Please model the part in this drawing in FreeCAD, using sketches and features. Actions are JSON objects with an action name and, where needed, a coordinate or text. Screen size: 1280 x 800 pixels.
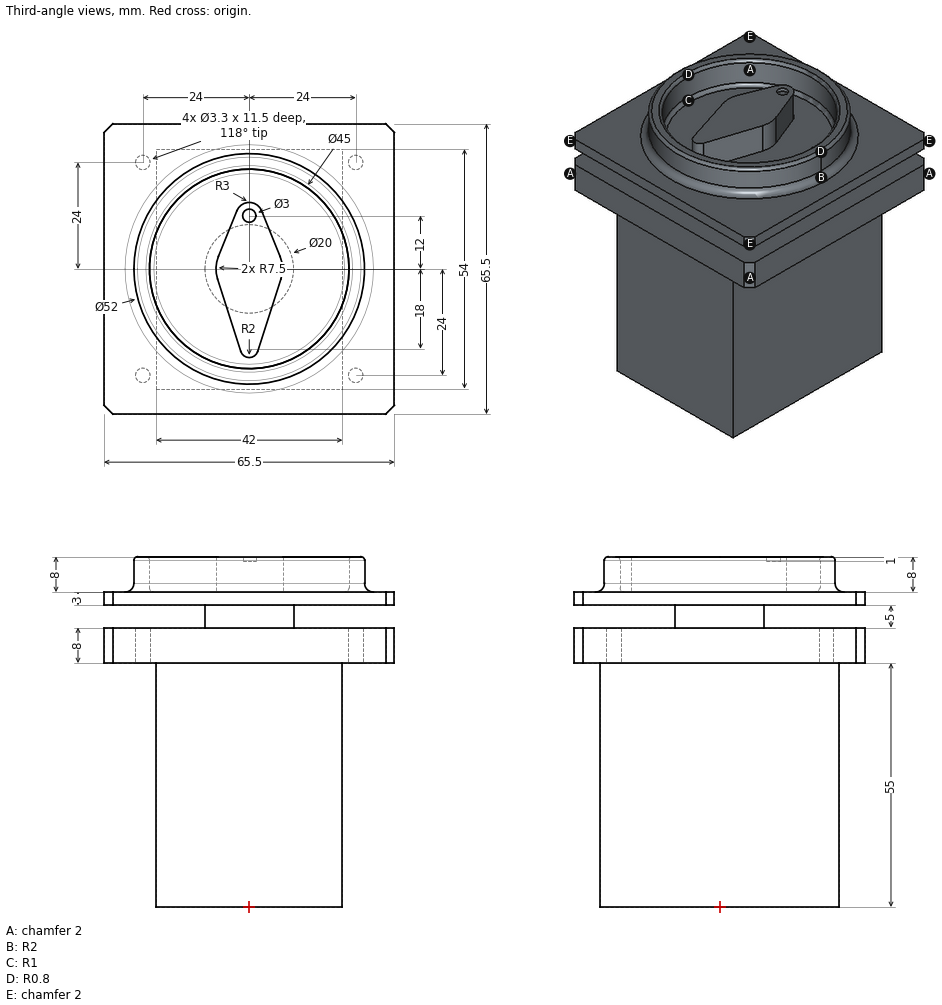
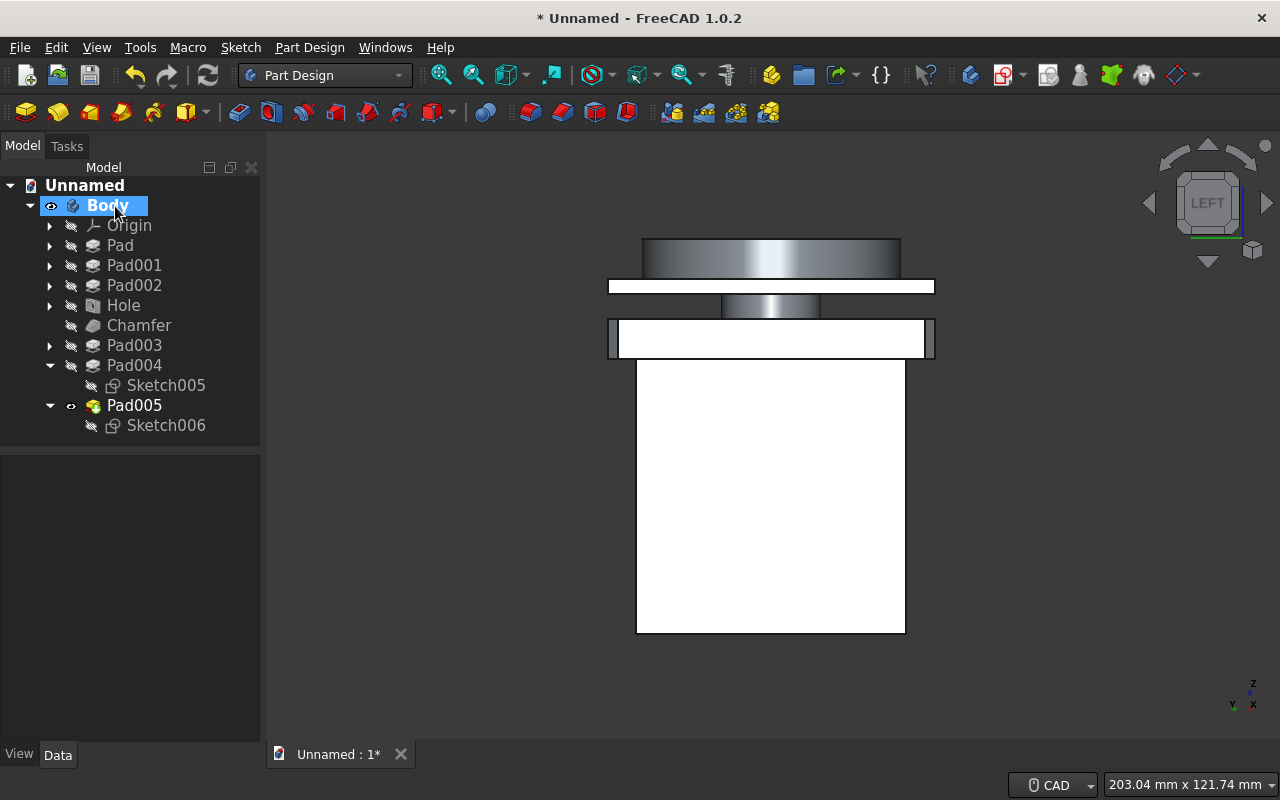
{"action": "key", "text": "v 3"}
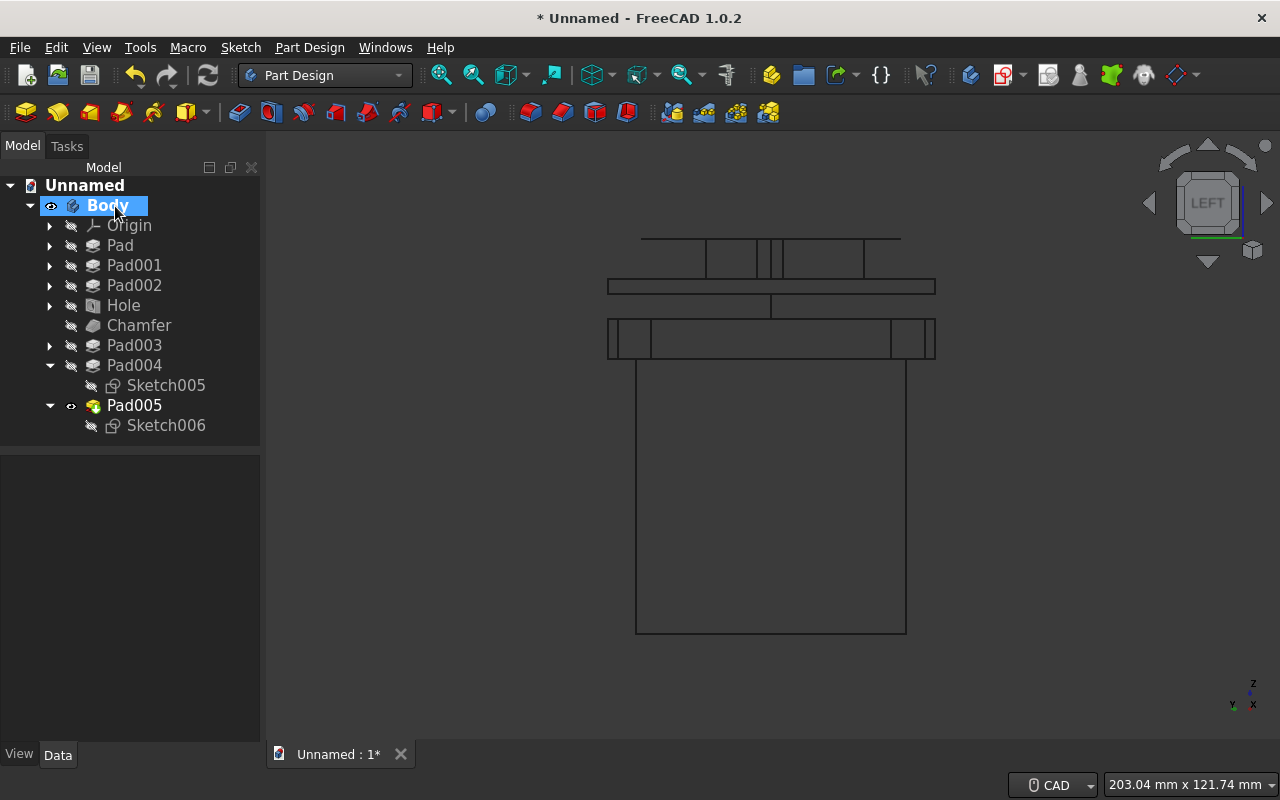
{"action": "key", "text": "0"}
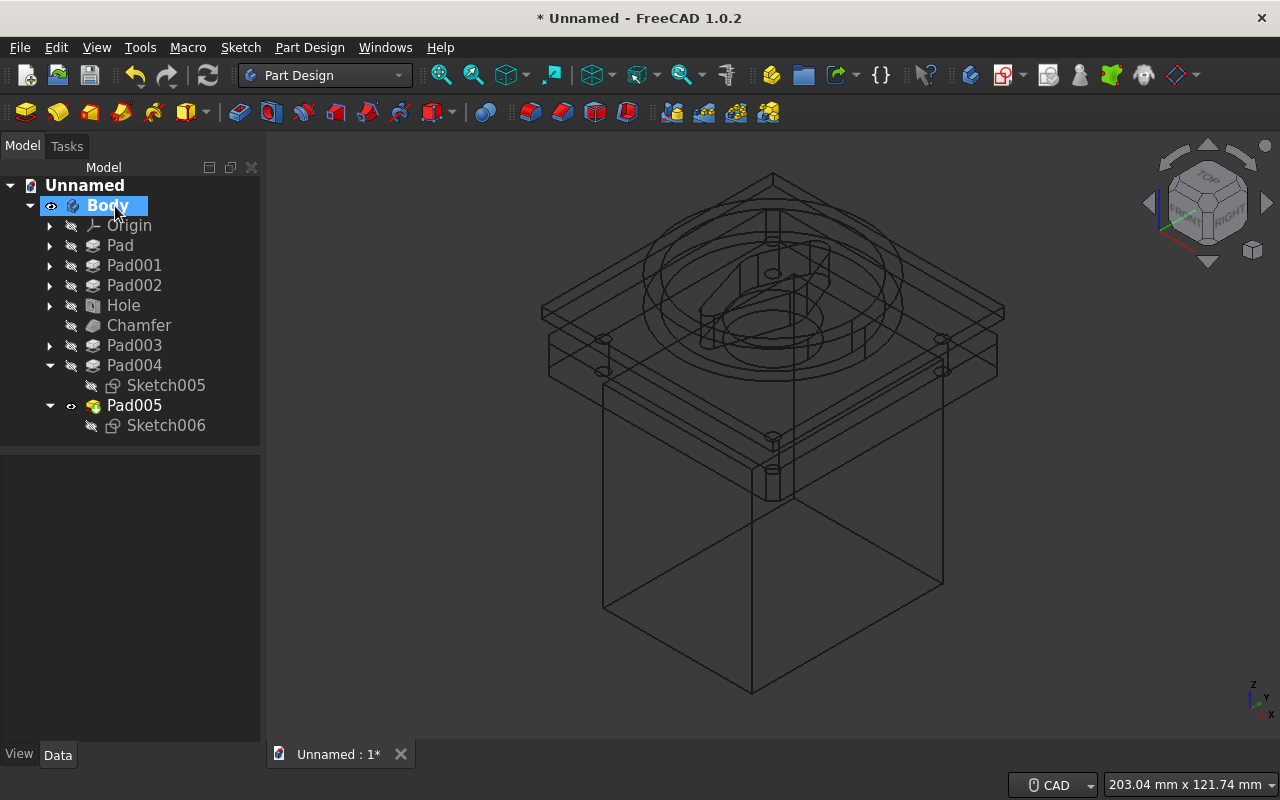
{"action": "left_click", "coordinate": [681, 252]}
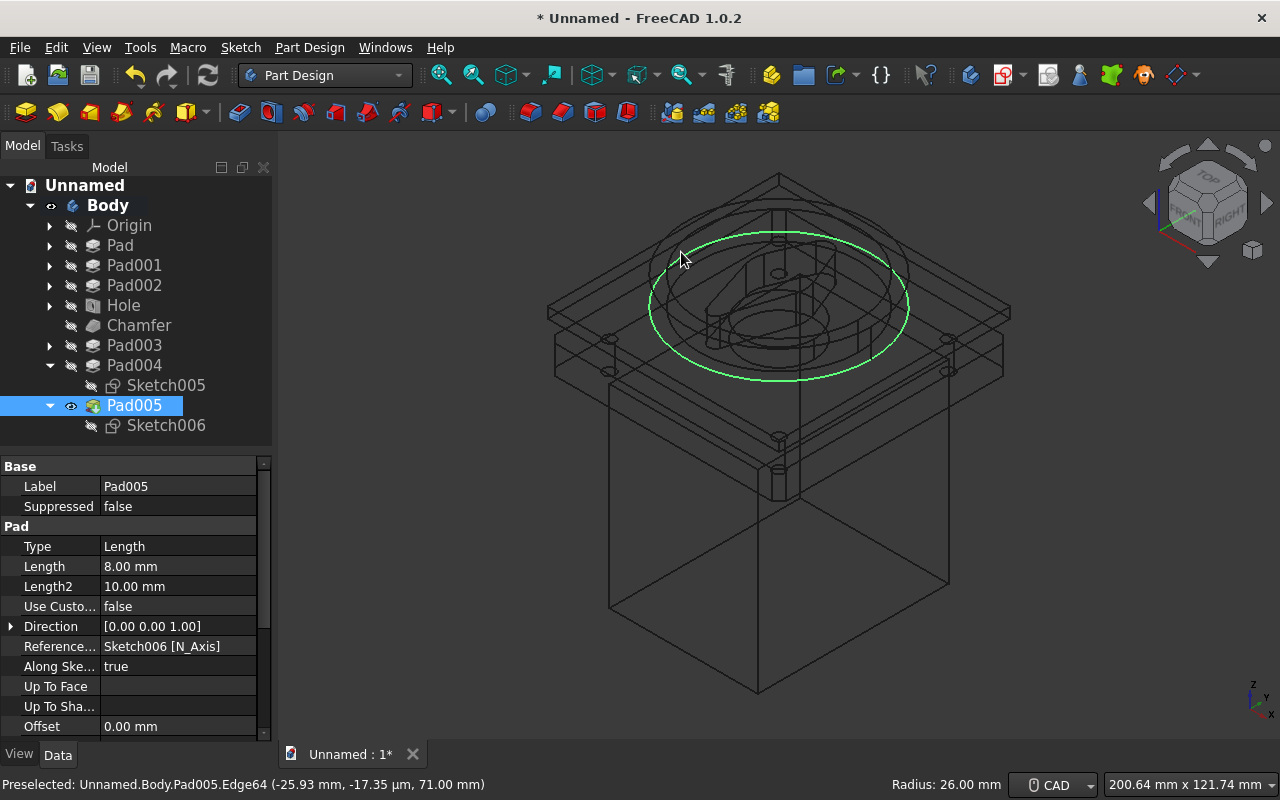
{"action": "key", "text": "v 1"}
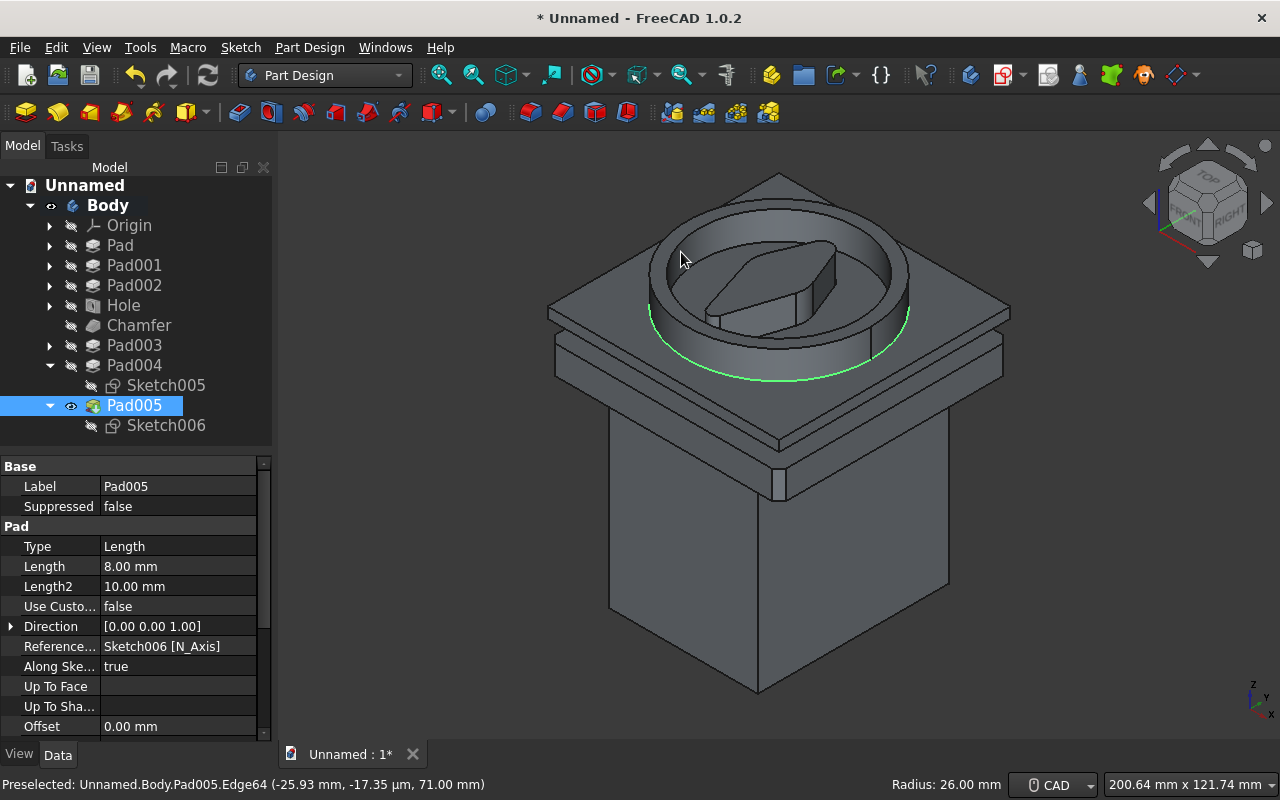
{"action": "left_click", "coordinate": [532, 112]}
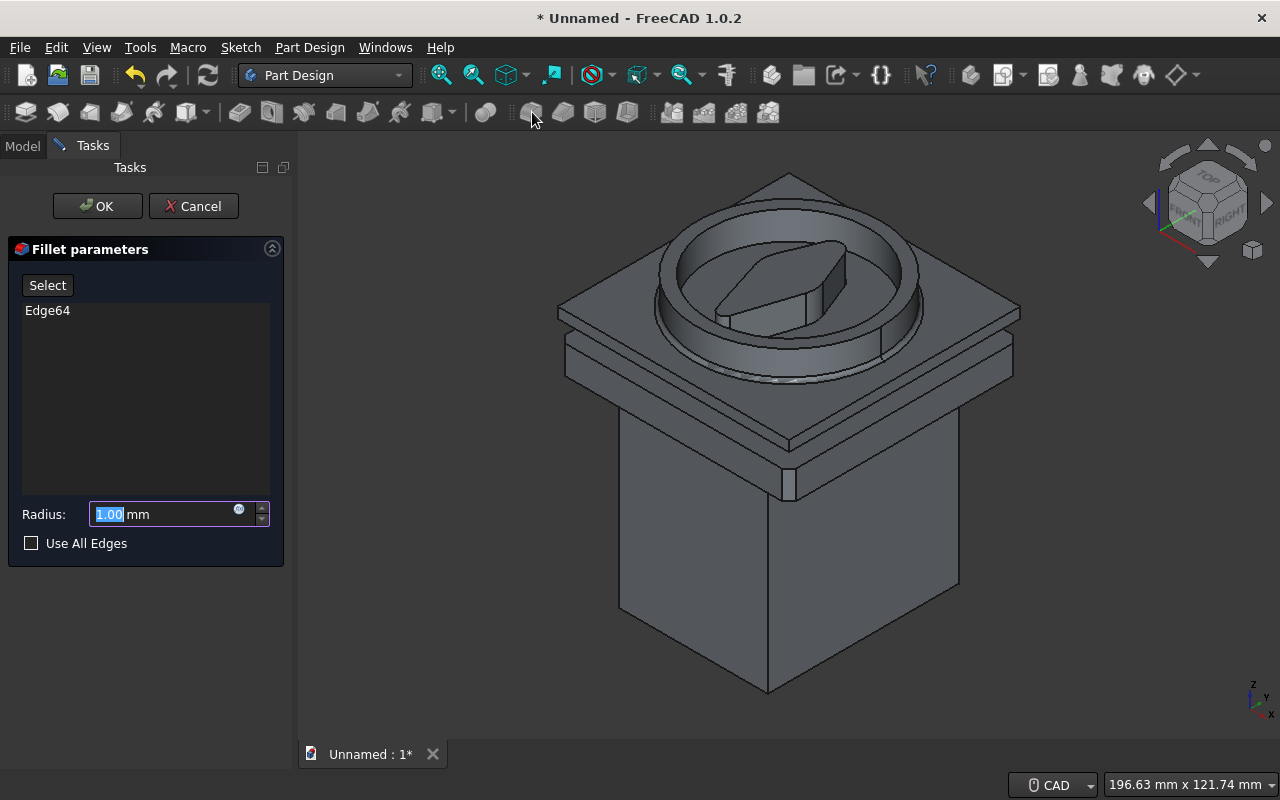
{"action": "type", "text": "2"}
{"action": "key", "text": "Tab"}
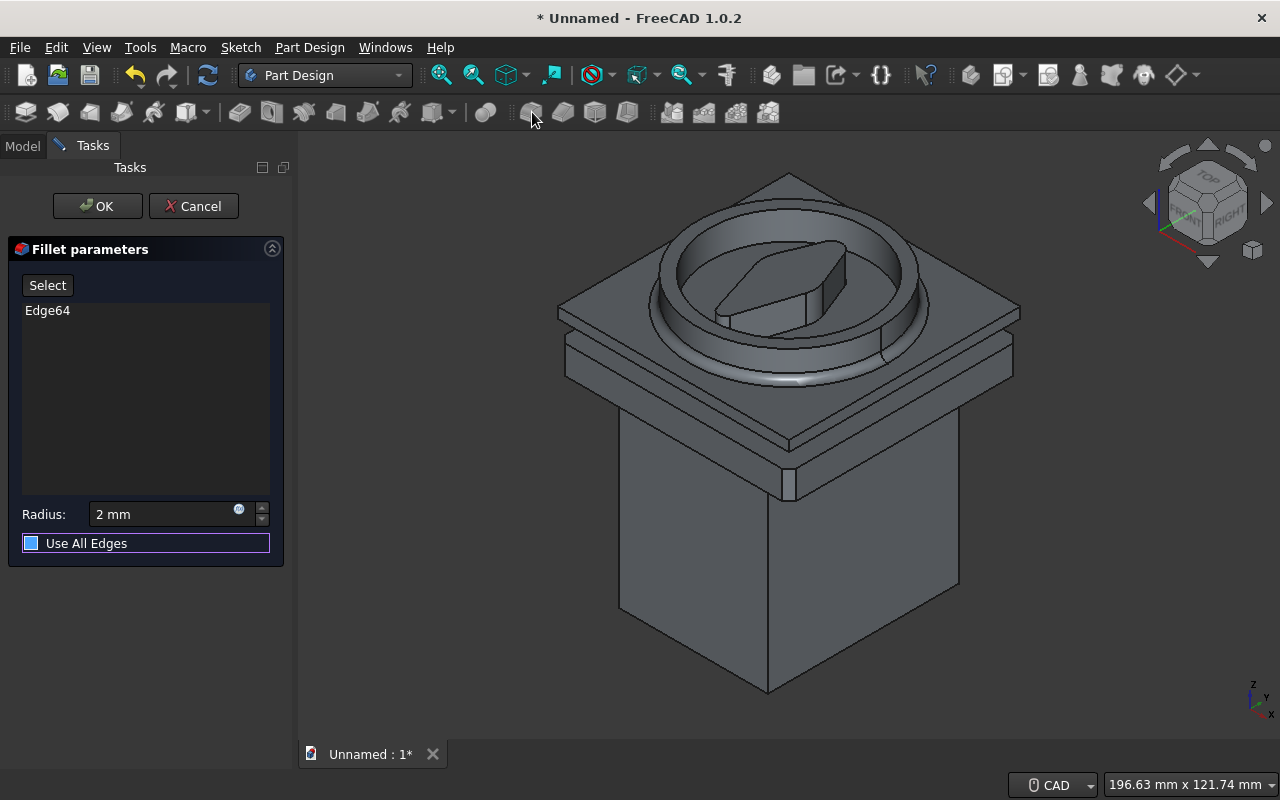
{"action": "left_click", "coordinate": [98, 206]}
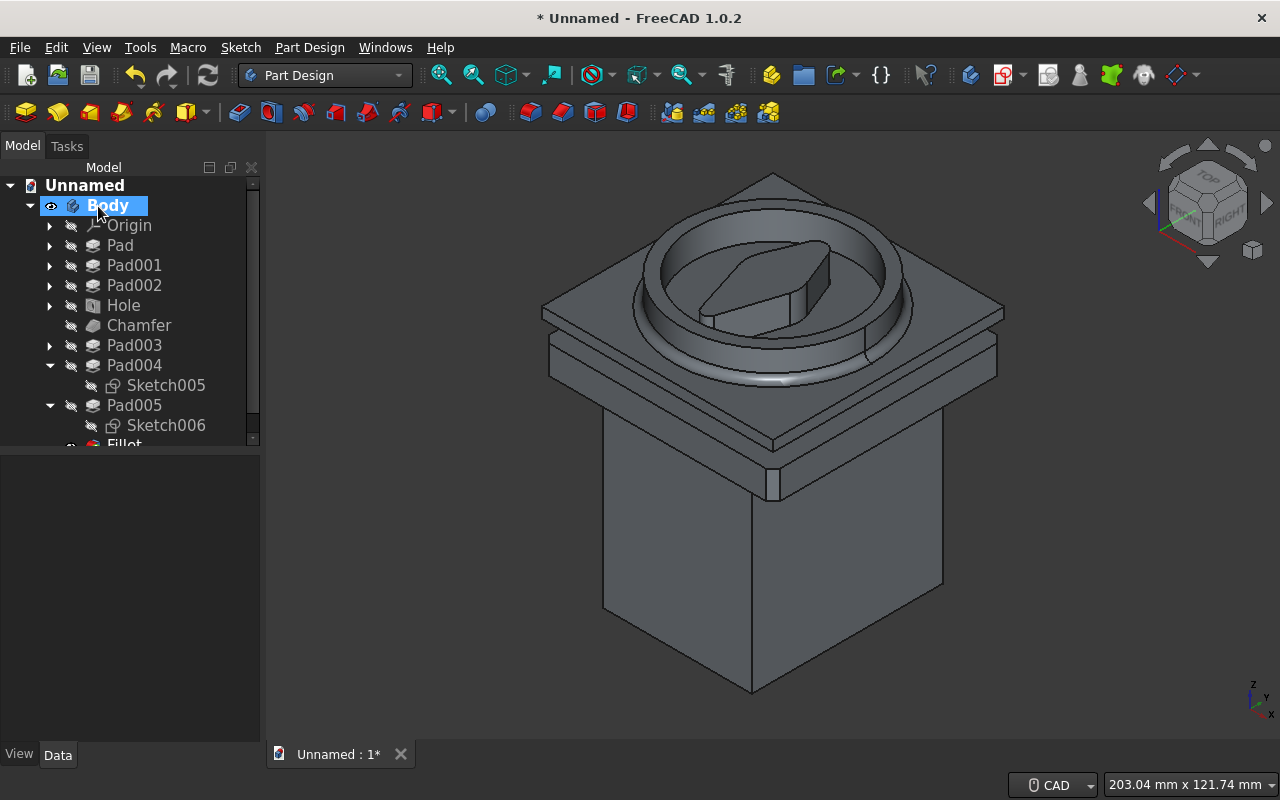
{"action": "key", "text": "2"}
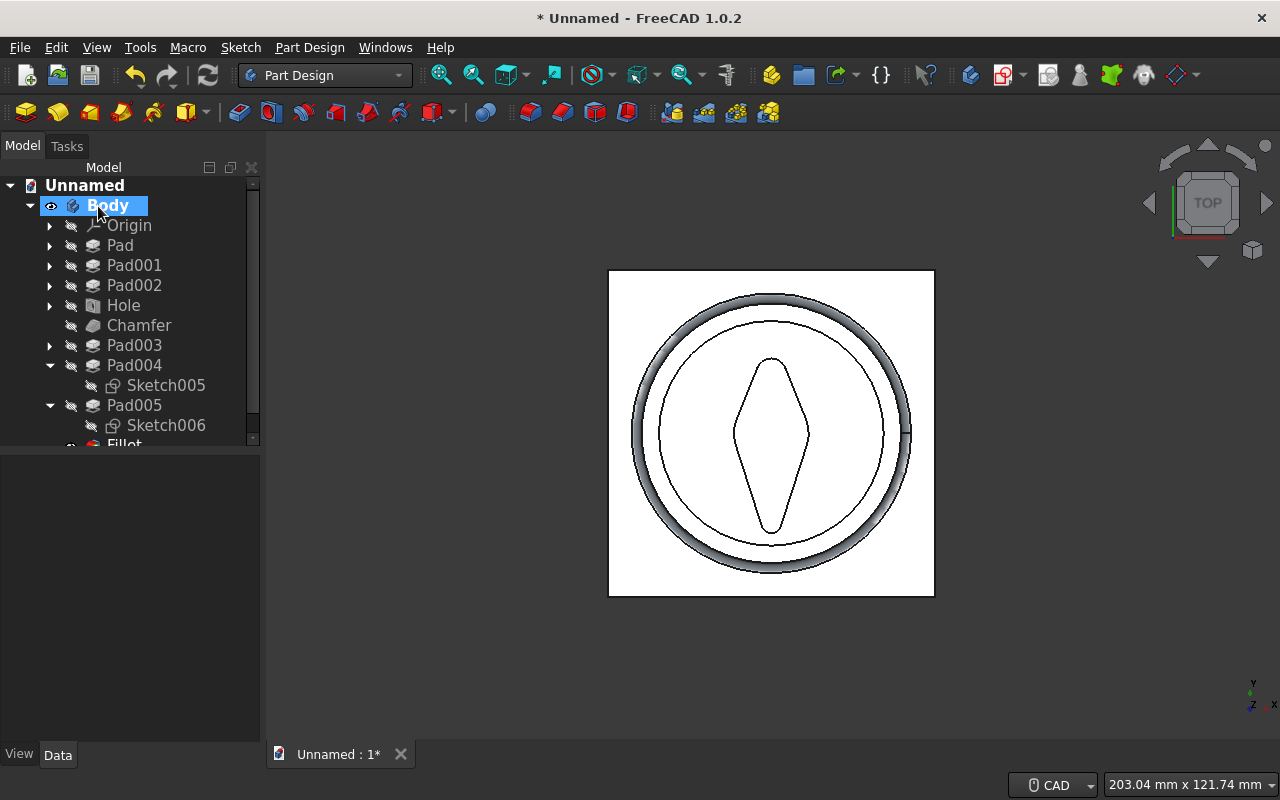
{"action": "key", "text": "0"}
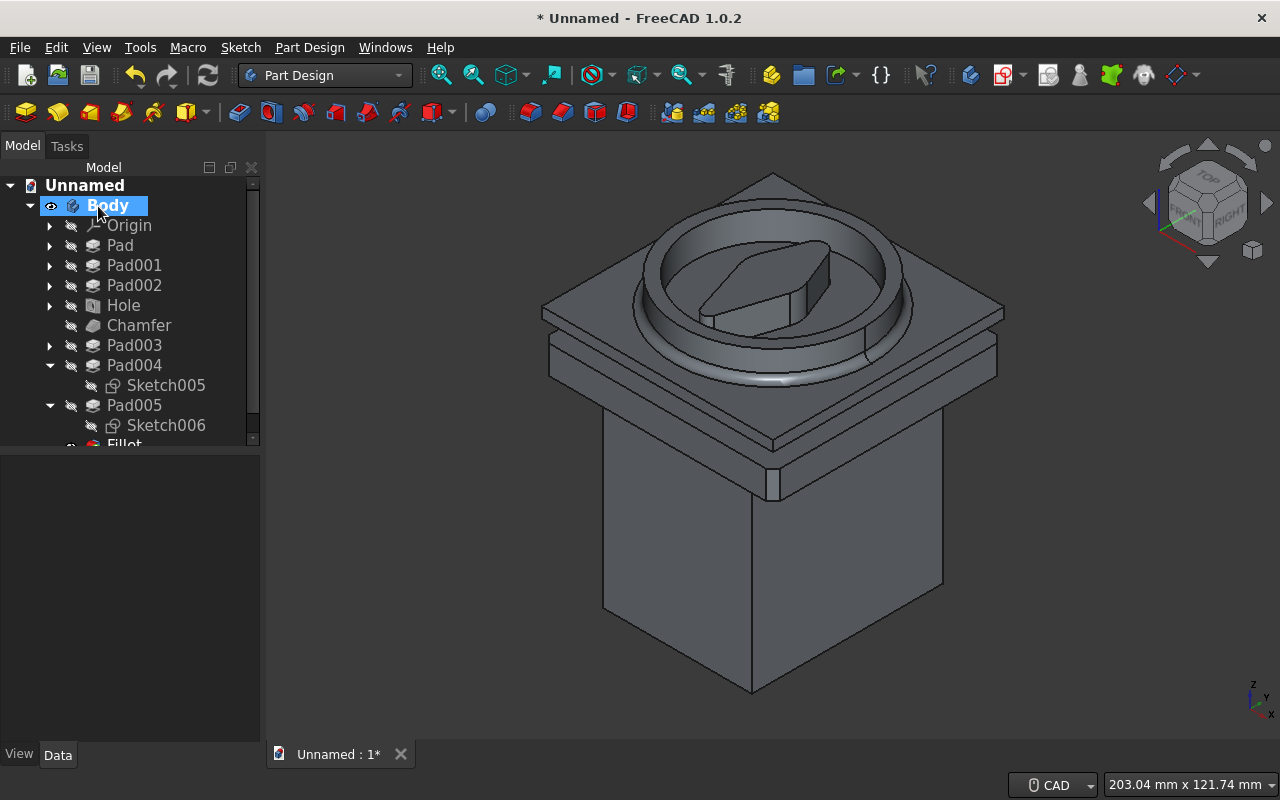
{"action": "key", "text": "1"}